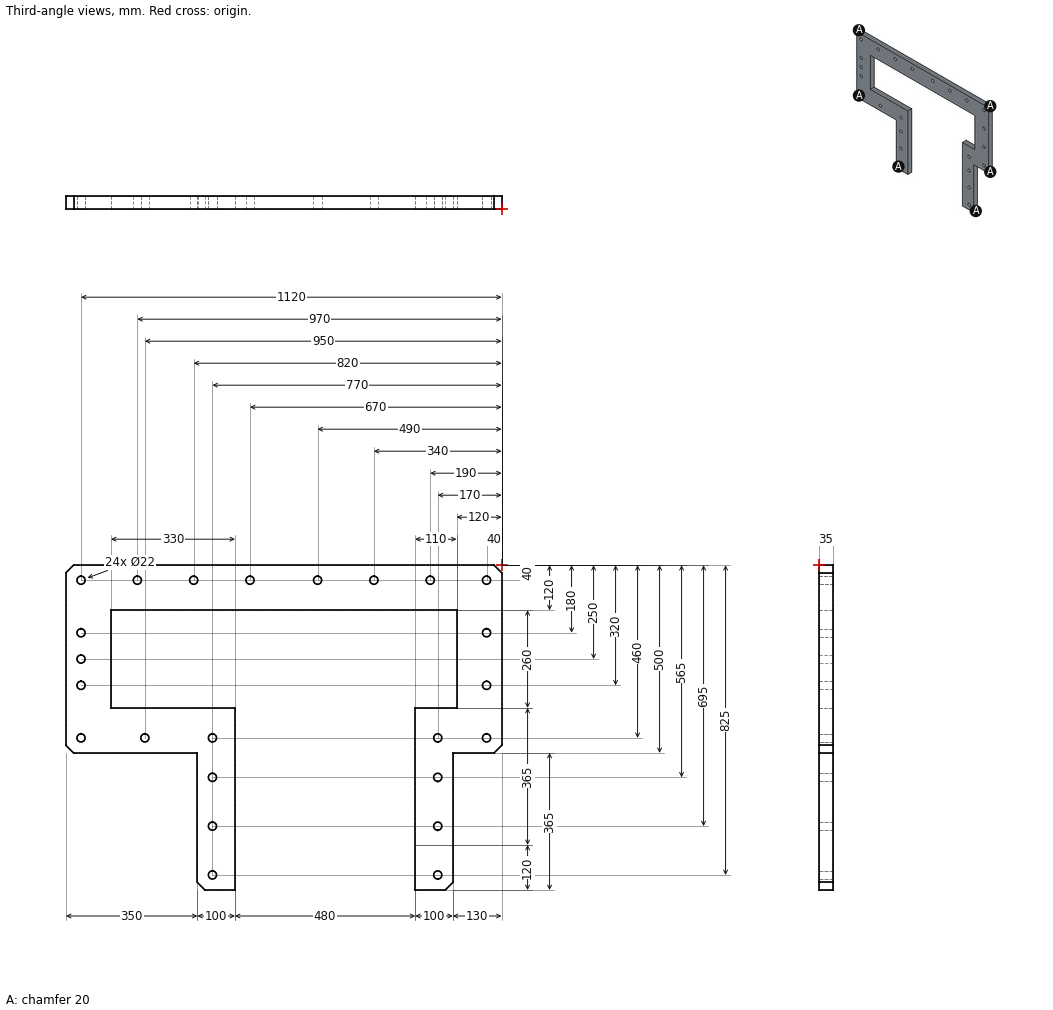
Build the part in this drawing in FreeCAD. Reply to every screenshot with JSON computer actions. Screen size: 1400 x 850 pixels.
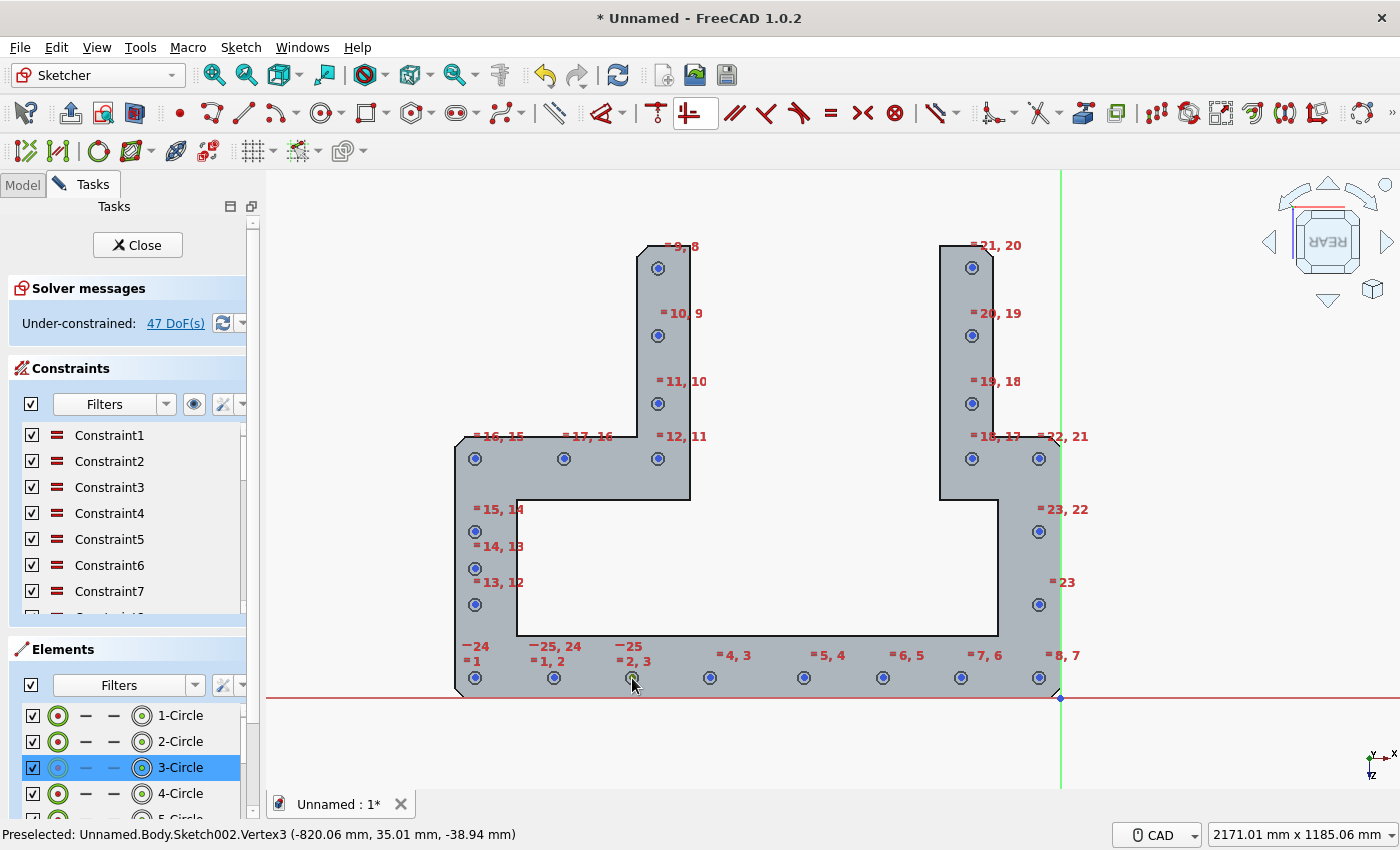
{"action": "left_click", "coordinate": [710, 678]}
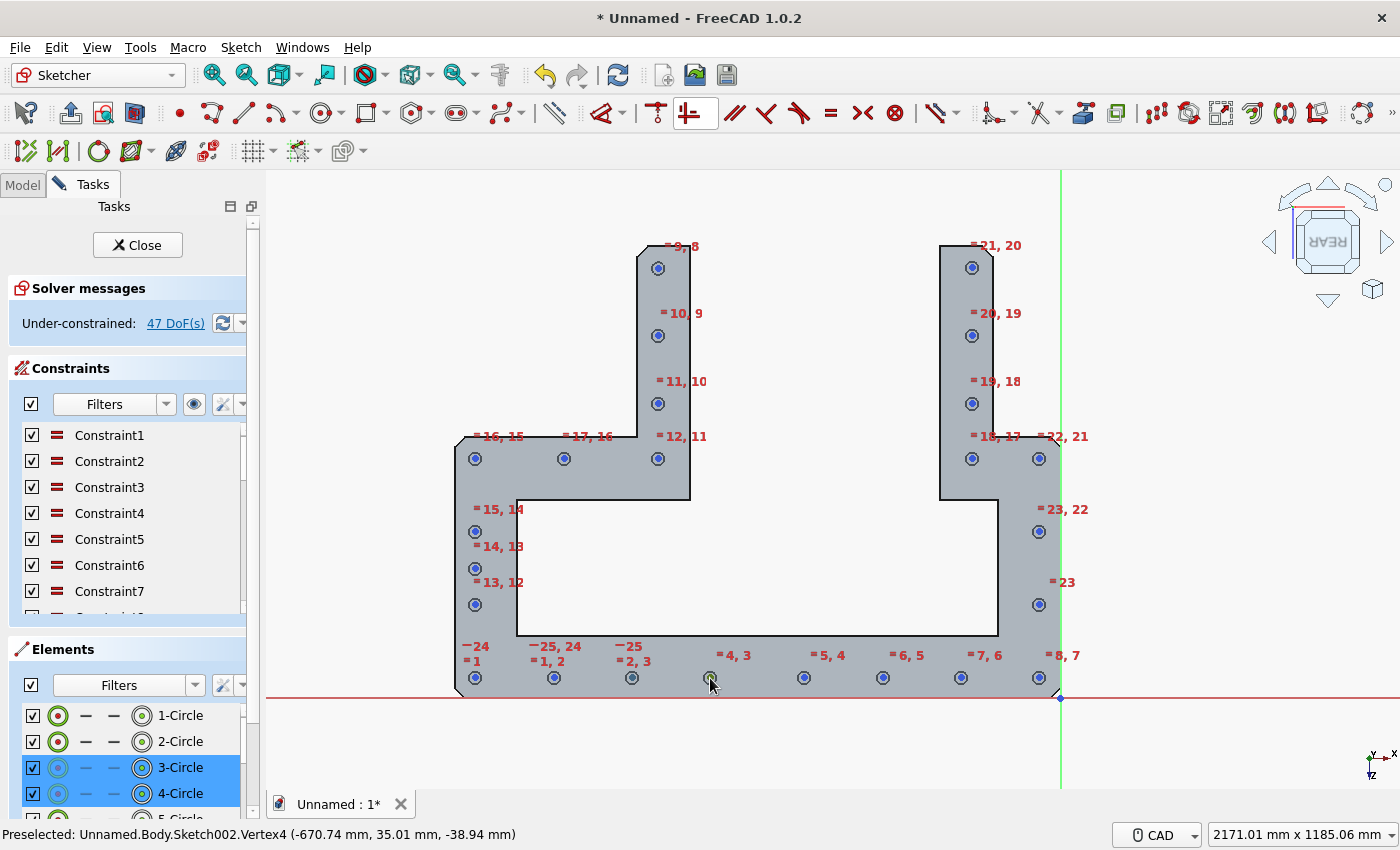
{"action": "key", "text": "h"}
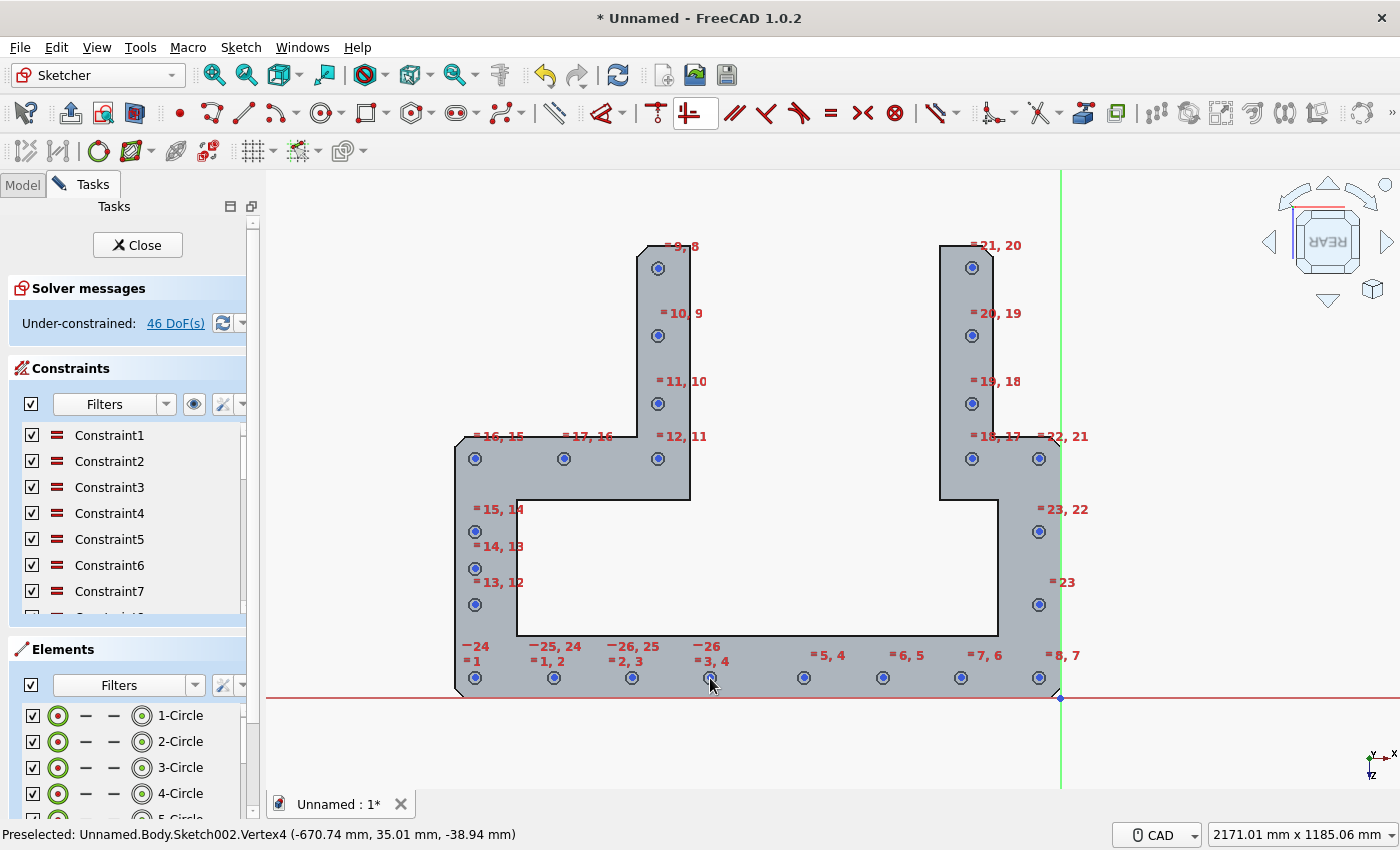
{"action": "left_click", "coordinate": [710, 678]}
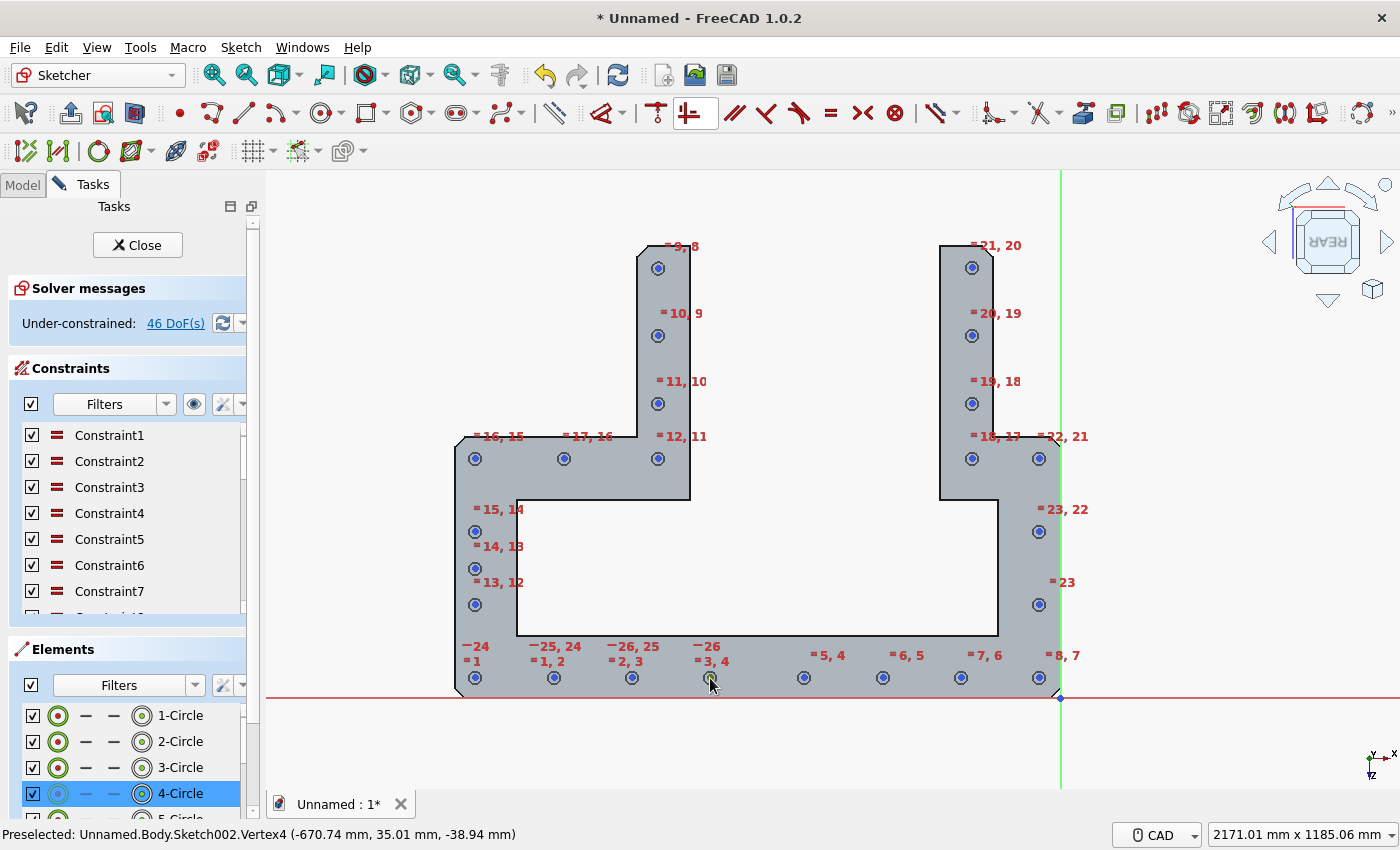
{"action": "left_click", "coordinate": [804, 678]}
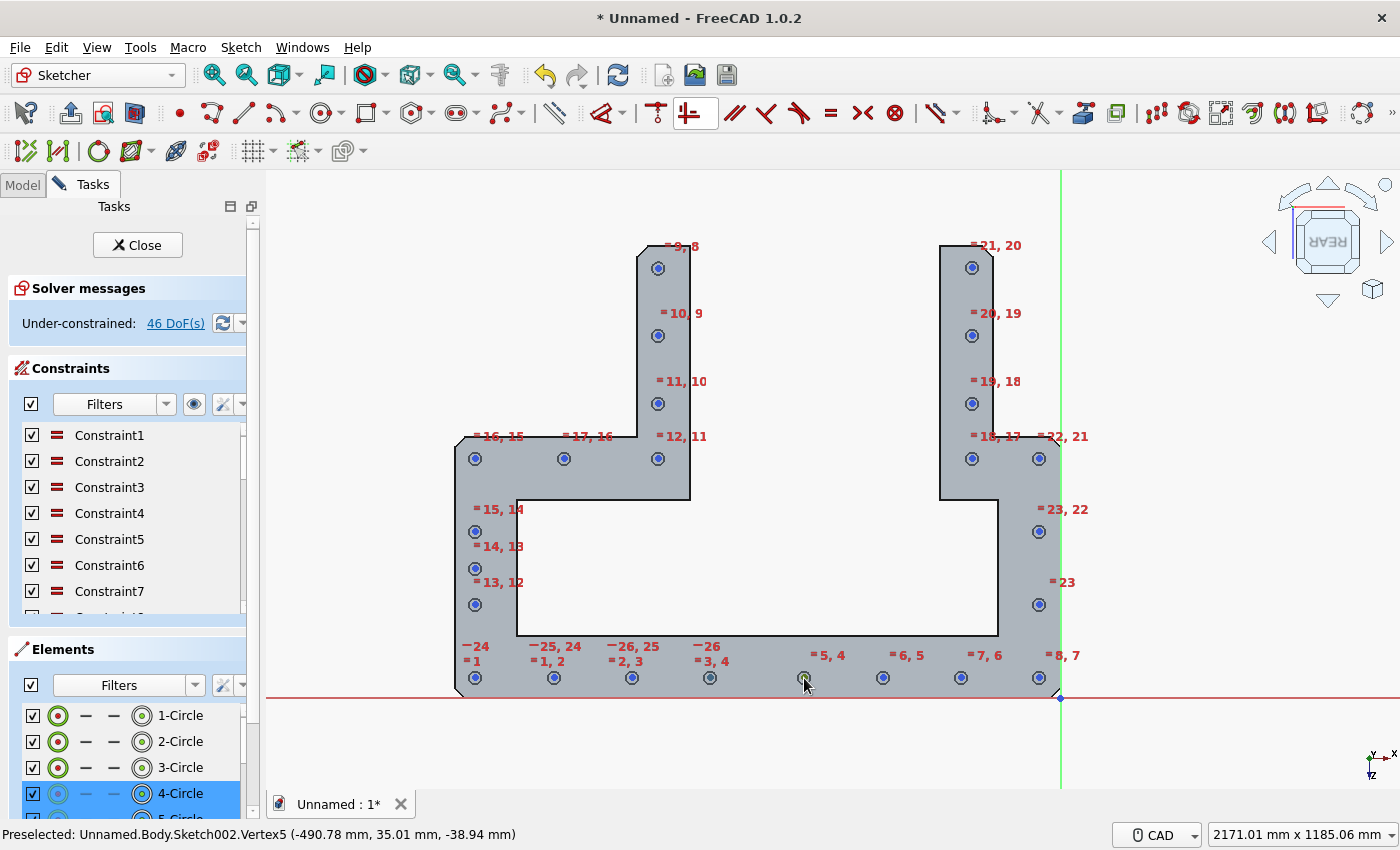
{"action": "key", "text": "h"}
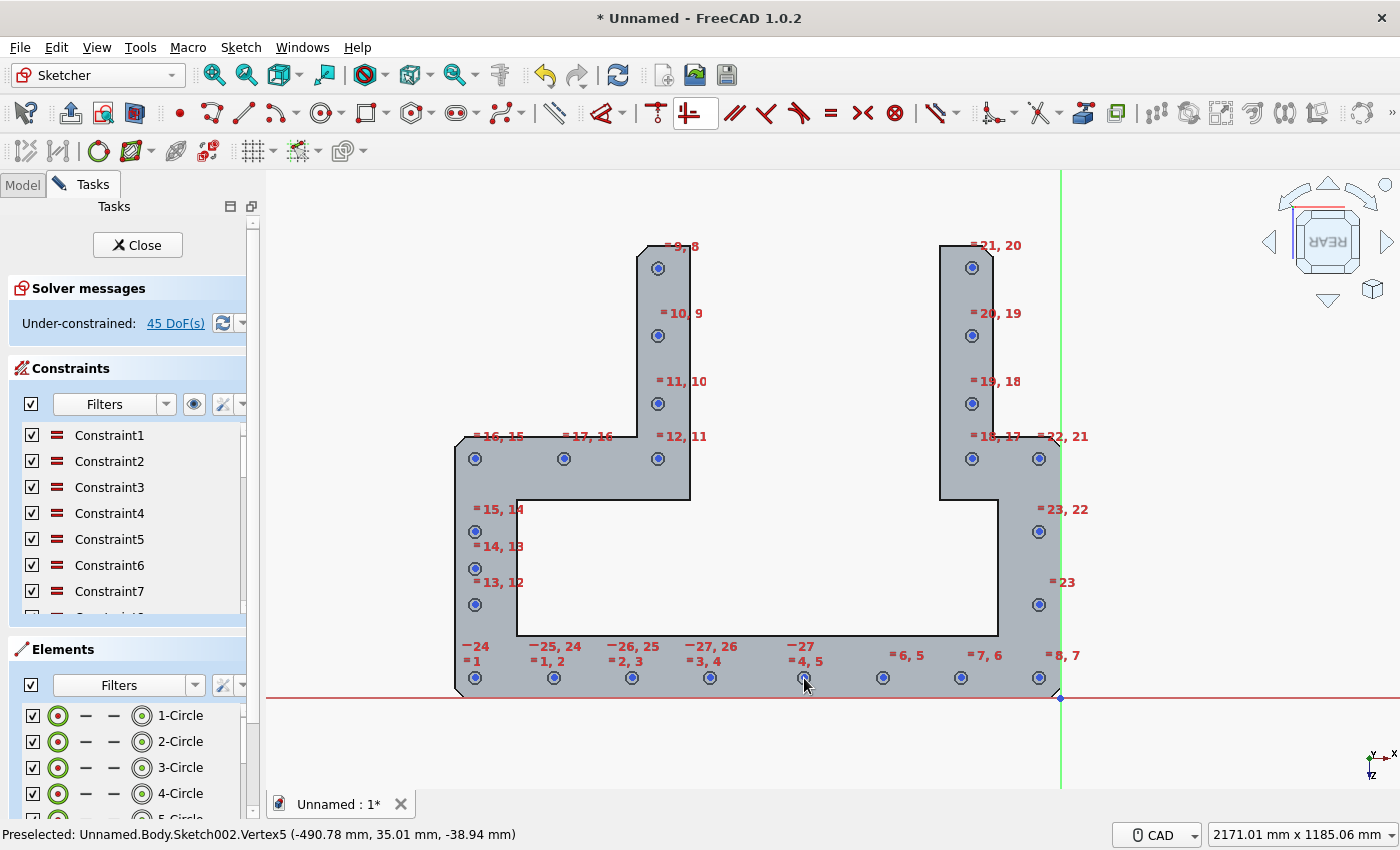
{"action": "left_click", "coordinate": [804, 678]}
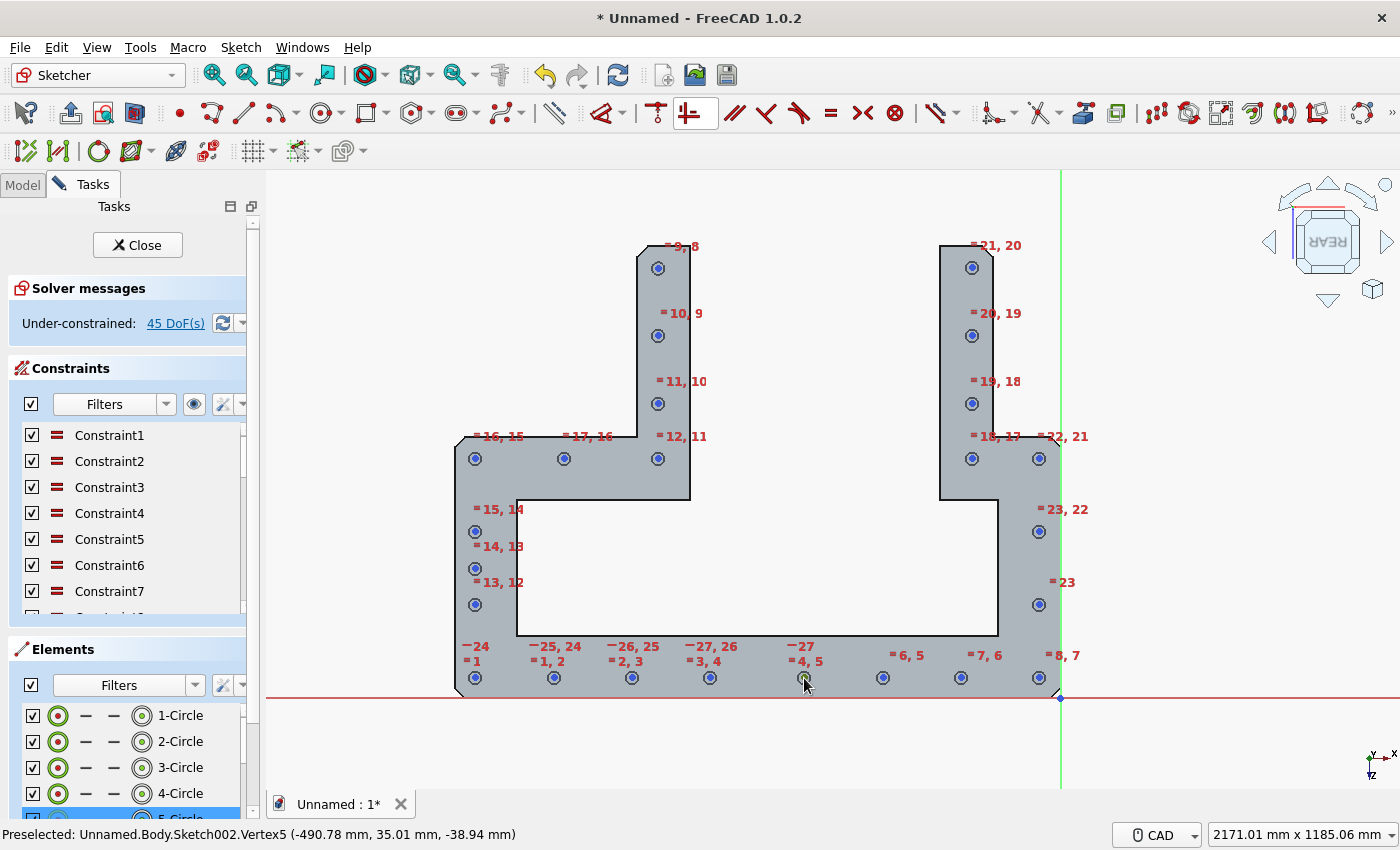
{"action": "left_click", "coordinate": [883, 678]}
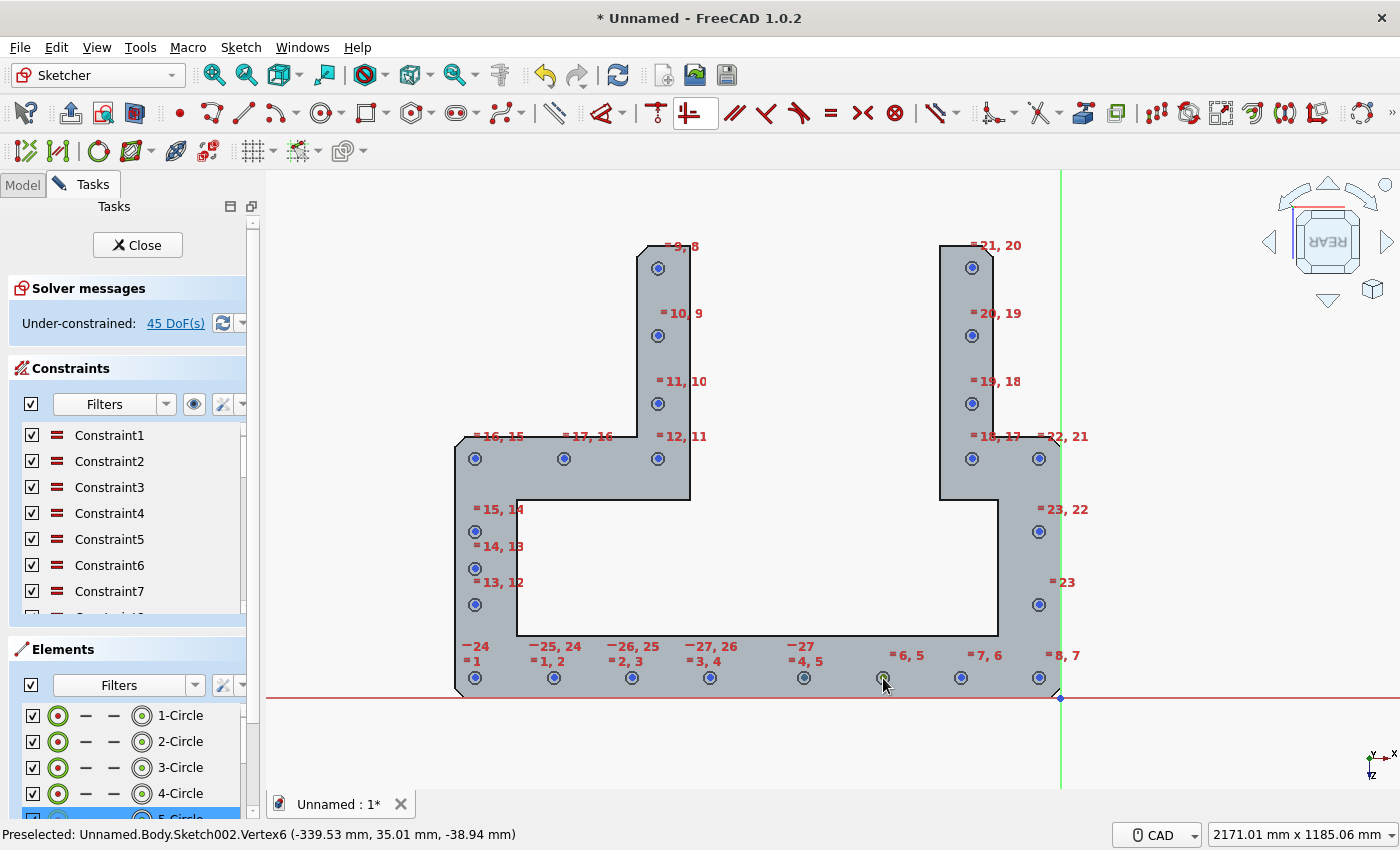
{"action": "key", "text": "h"}